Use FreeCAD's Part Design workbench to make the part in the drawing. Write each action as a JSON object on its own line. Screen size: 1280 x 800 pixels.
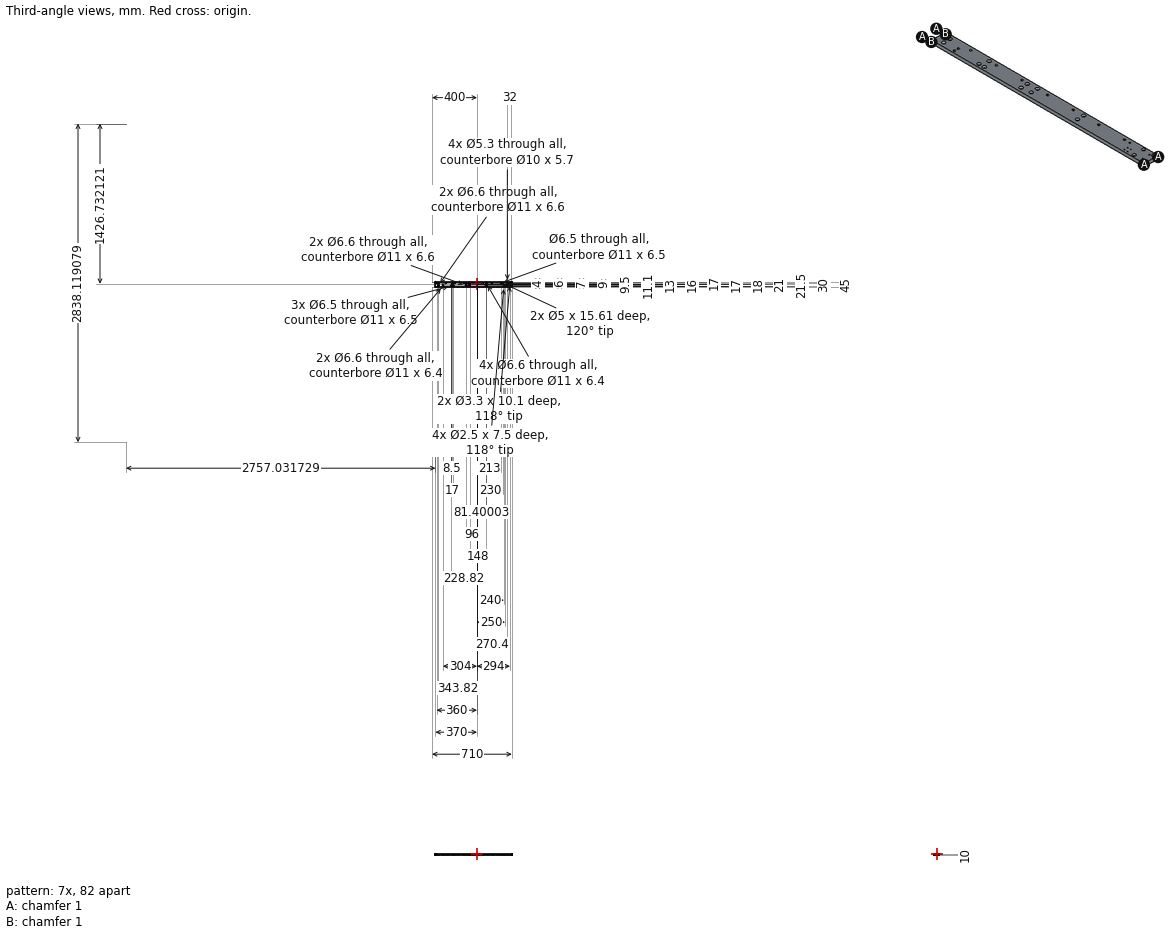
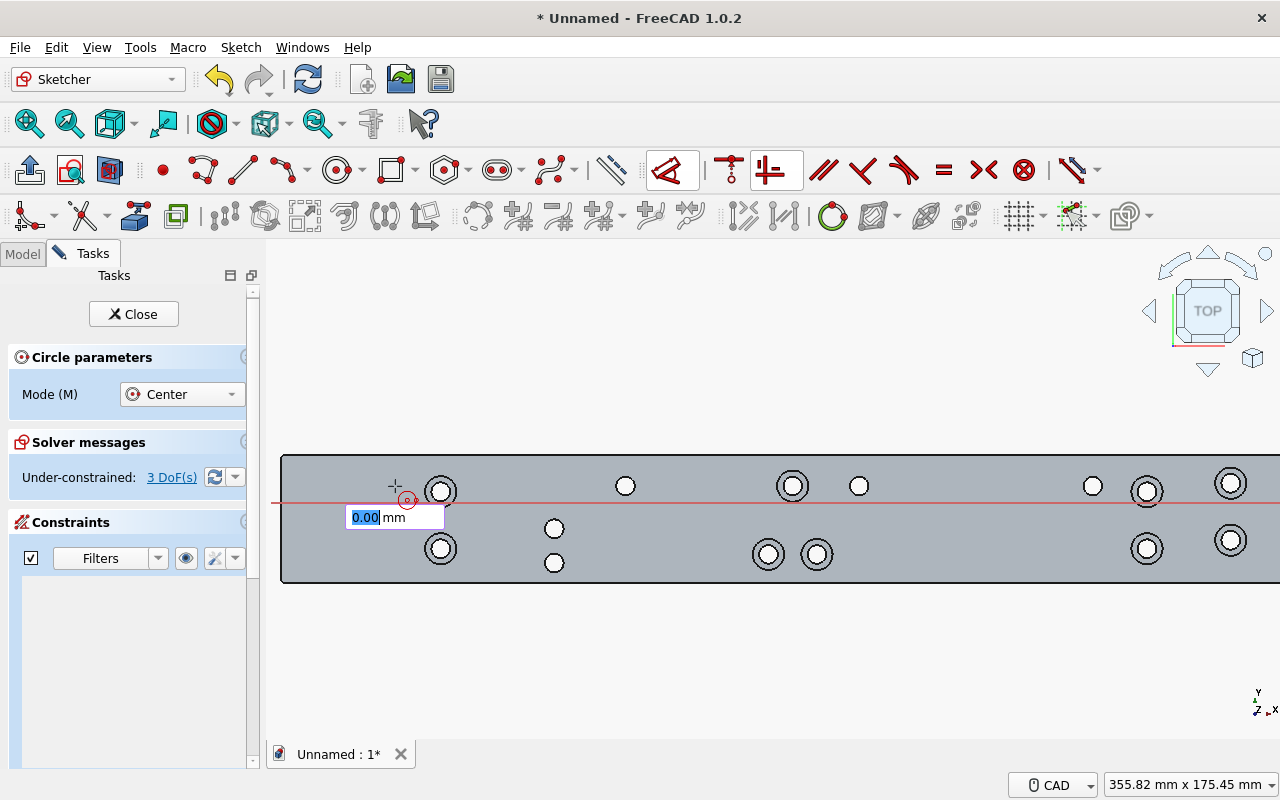
{"action": "scroll", "coordinate": [400, 481], "scroll_direction": "up", "scroll_amount": 5}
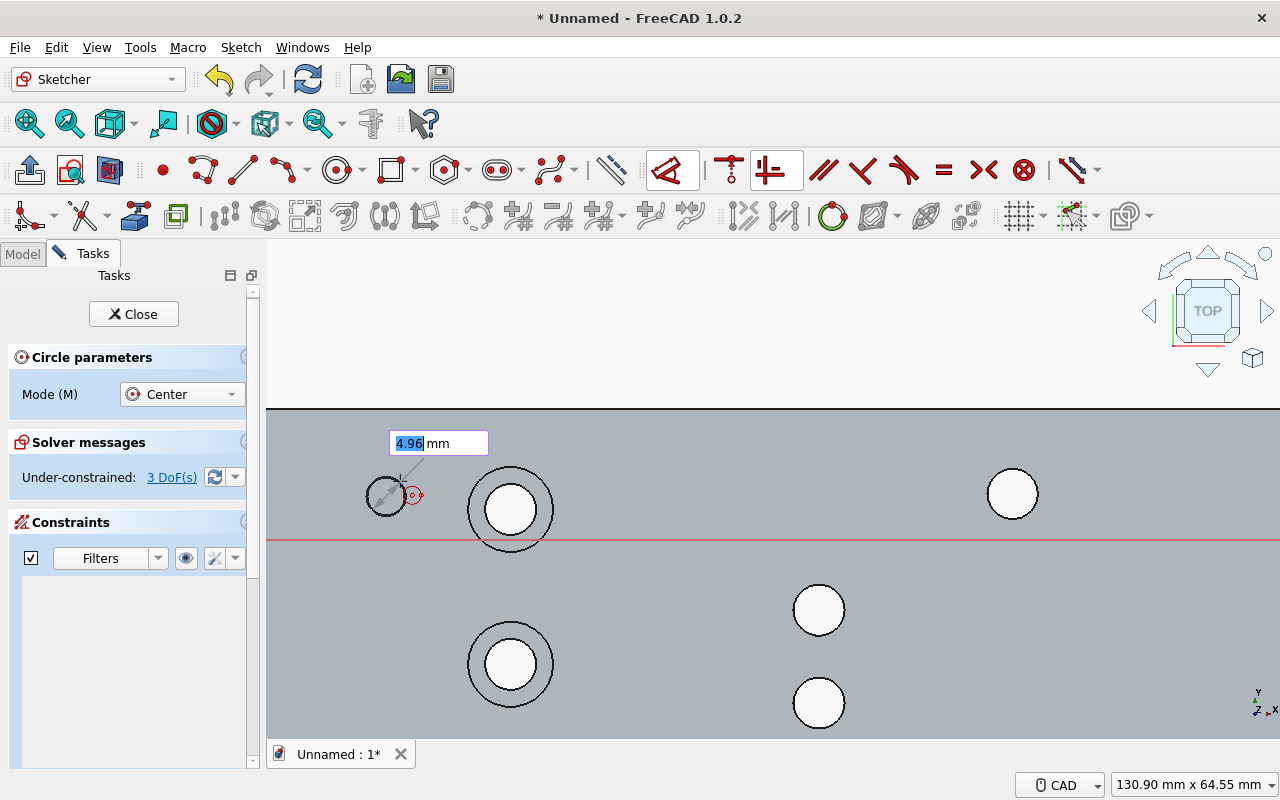
{"action": "left_click", "coordinate": [399, 480]}
{"action": "key", "text": "Escape"}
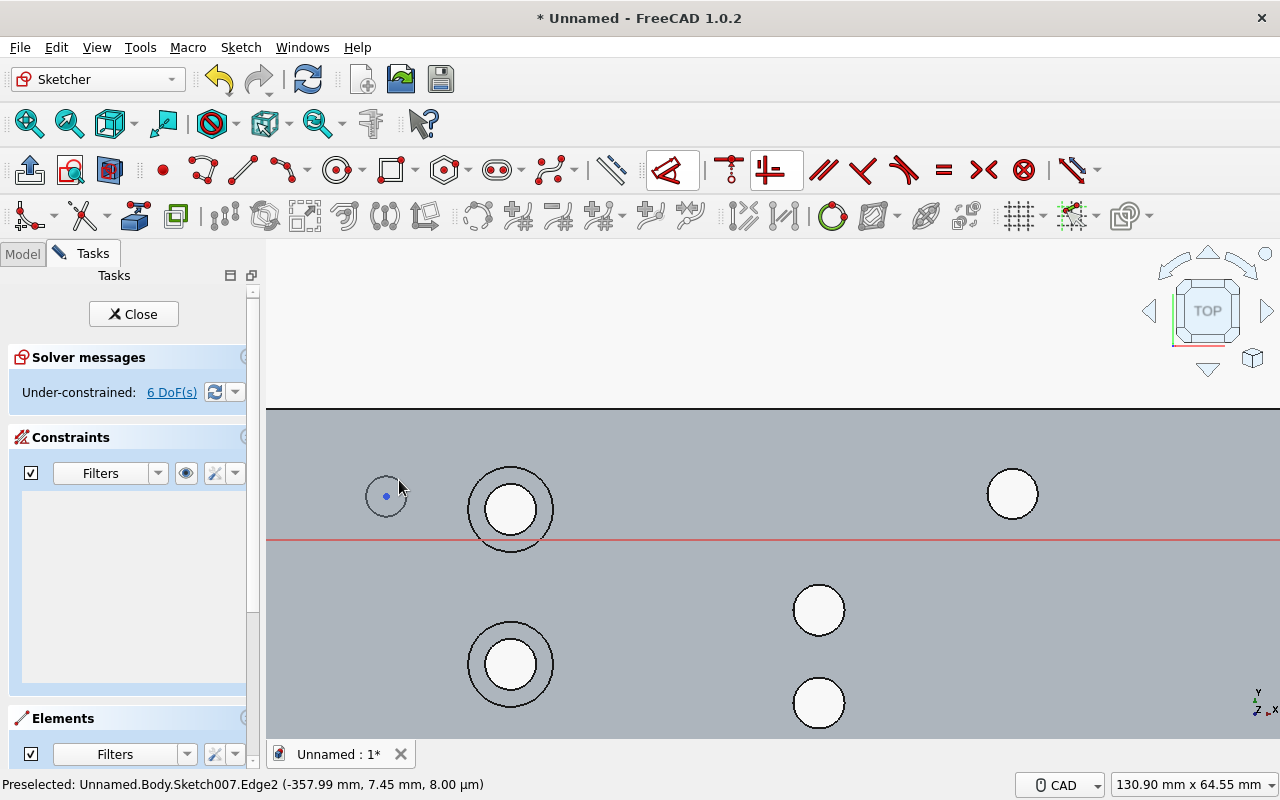
{"action": "scroll", "coordinate": [397, 486], "scroll_direction": "down", "scroll_amount": 10}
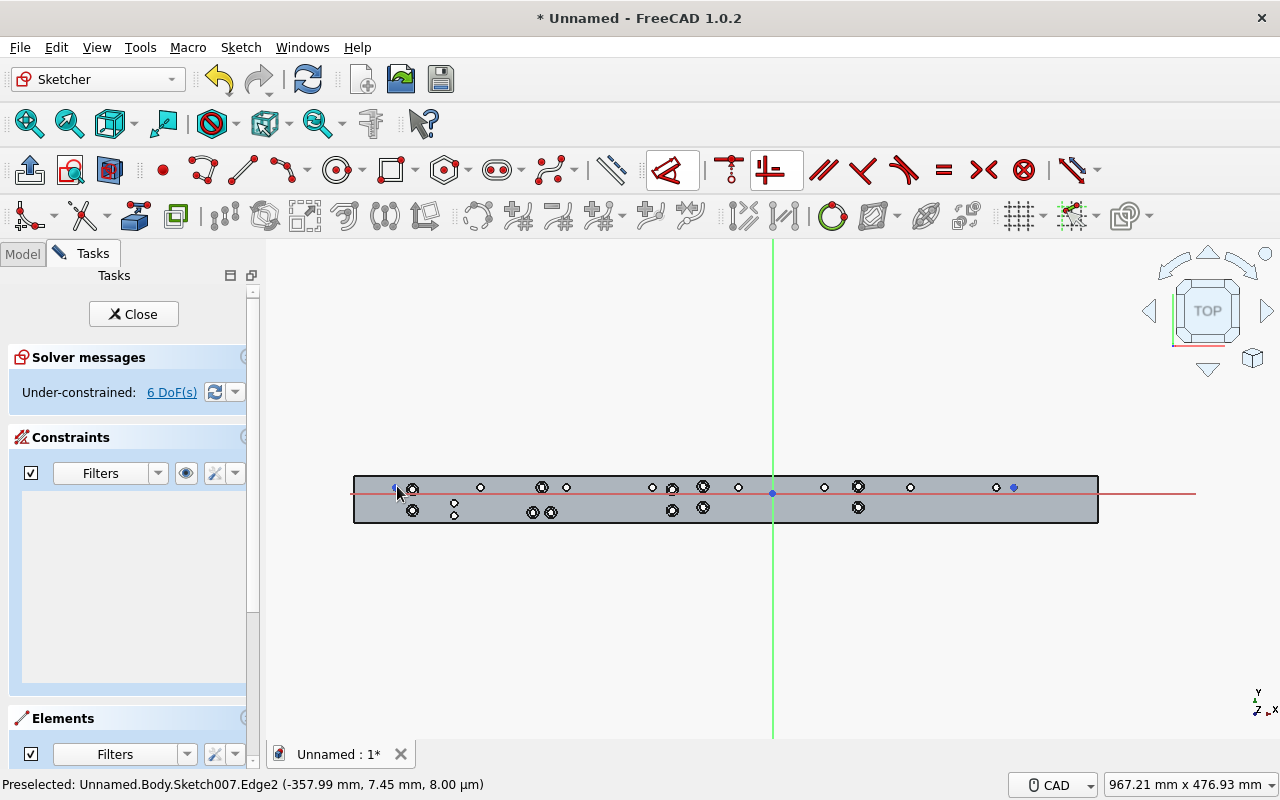
{"action": "scroll", "coordinate": [1016, 486], "scroll_direction": "up", "scroll_amount": 8}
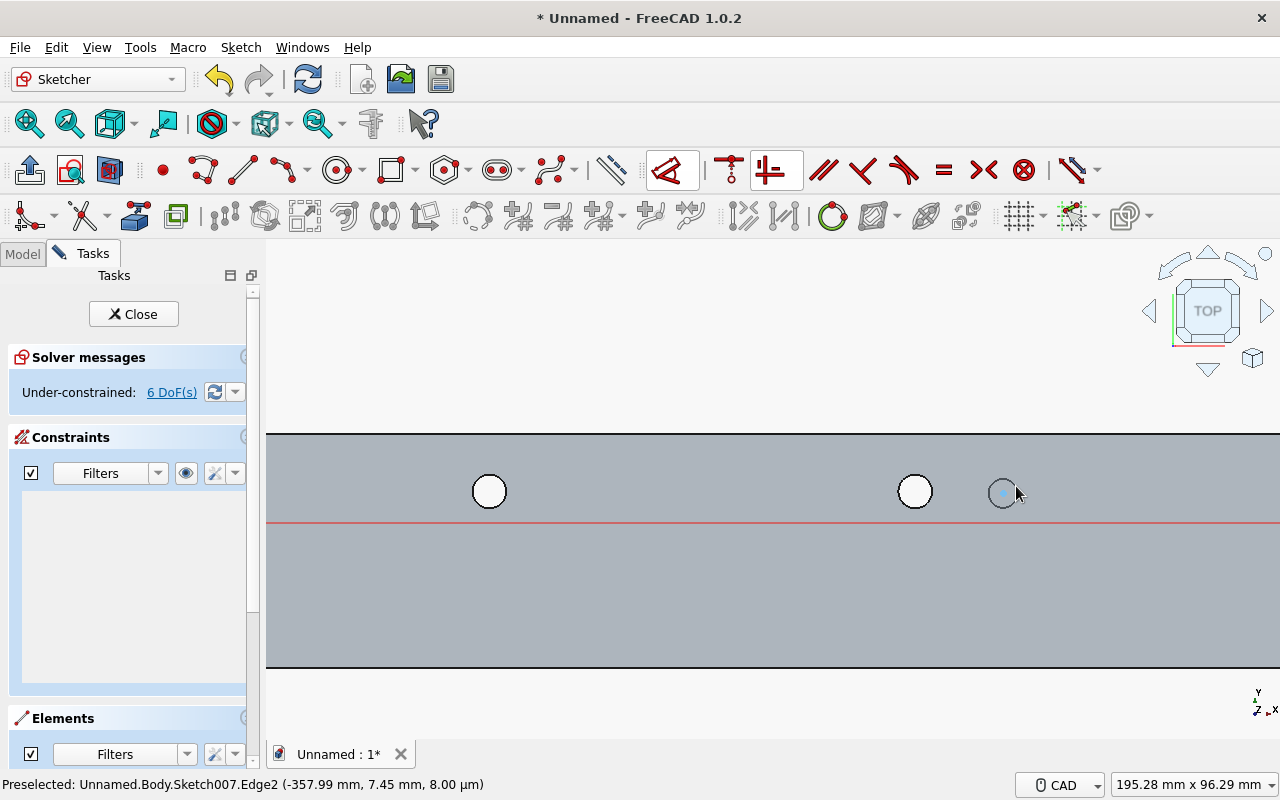
{"action": "left_click", "coordinate": [1013, 483]}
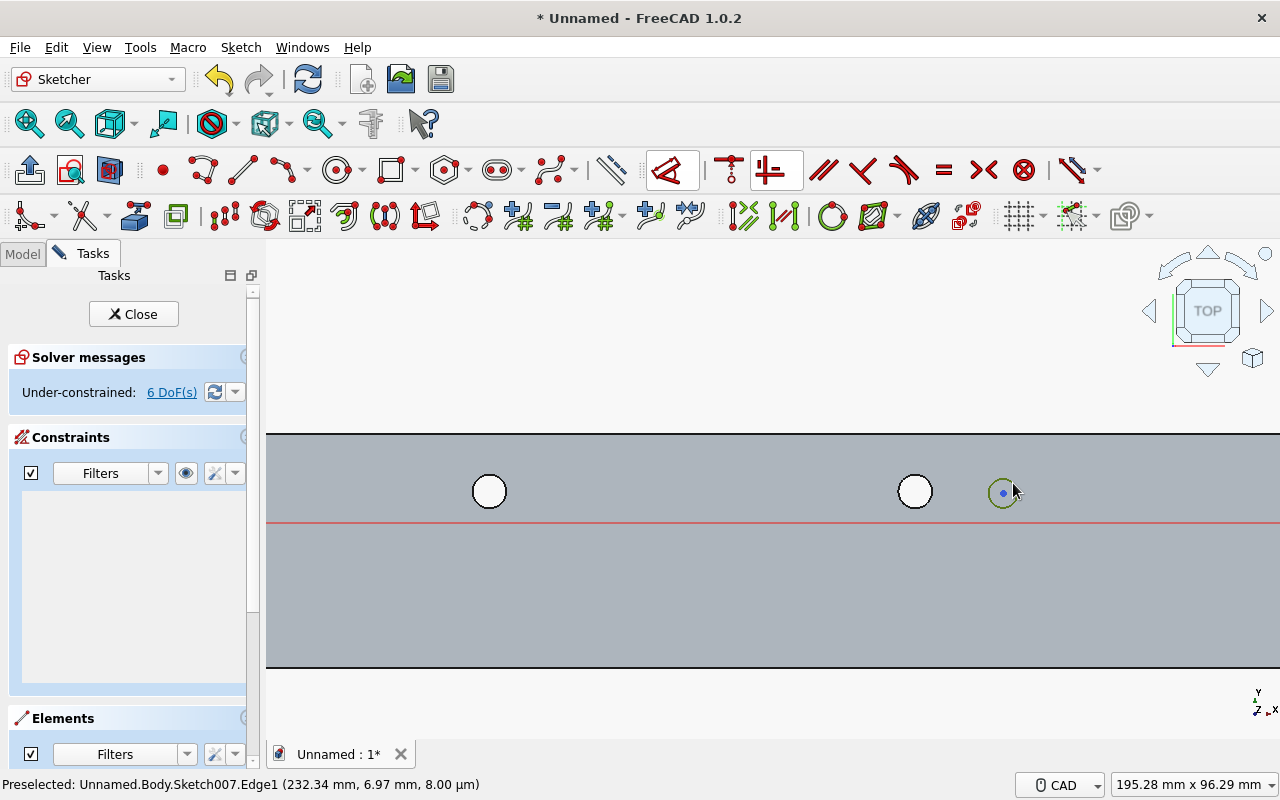
{"action": "scroll", "coordinate": [1016, 486], "scroll_direction": "down", "scroll_amount": 8}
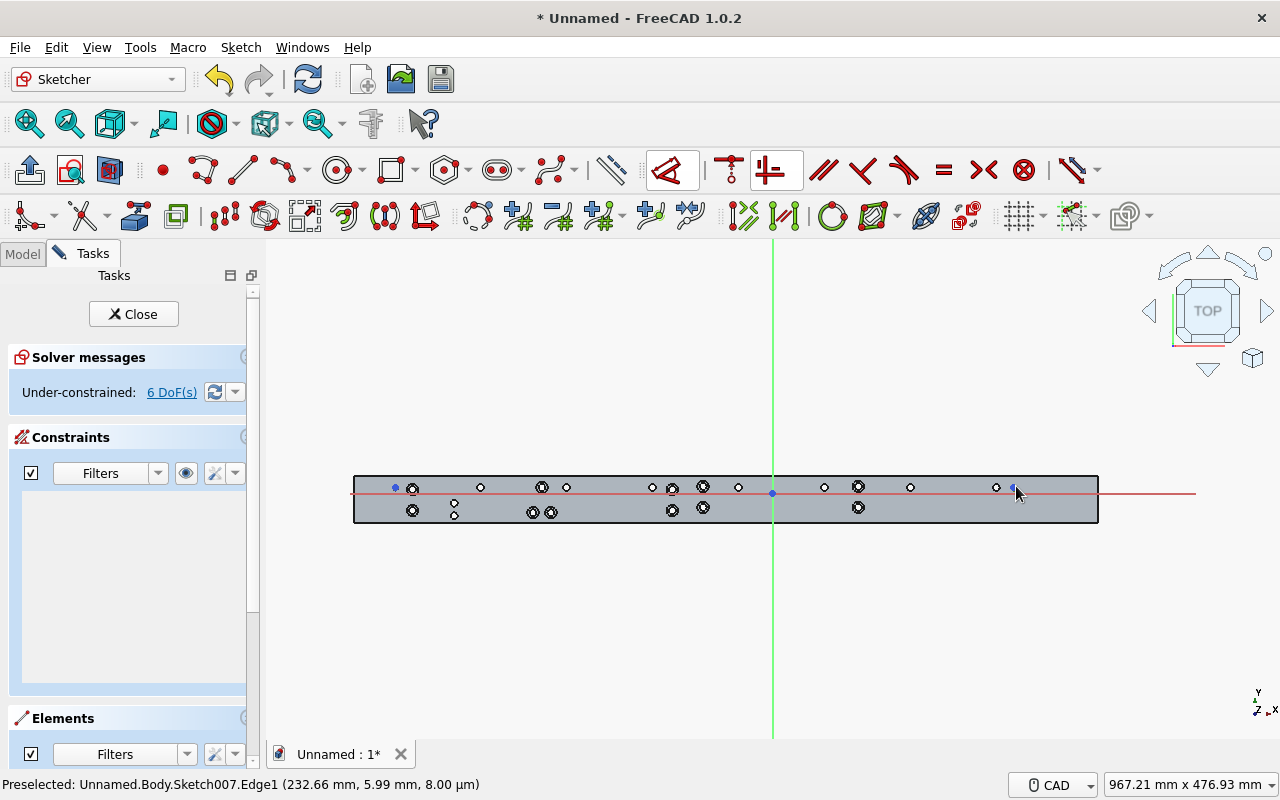
{"action": "scroll", "coordinate": [398, 486], "scroll_direction": "up", "scroll_amount": 9}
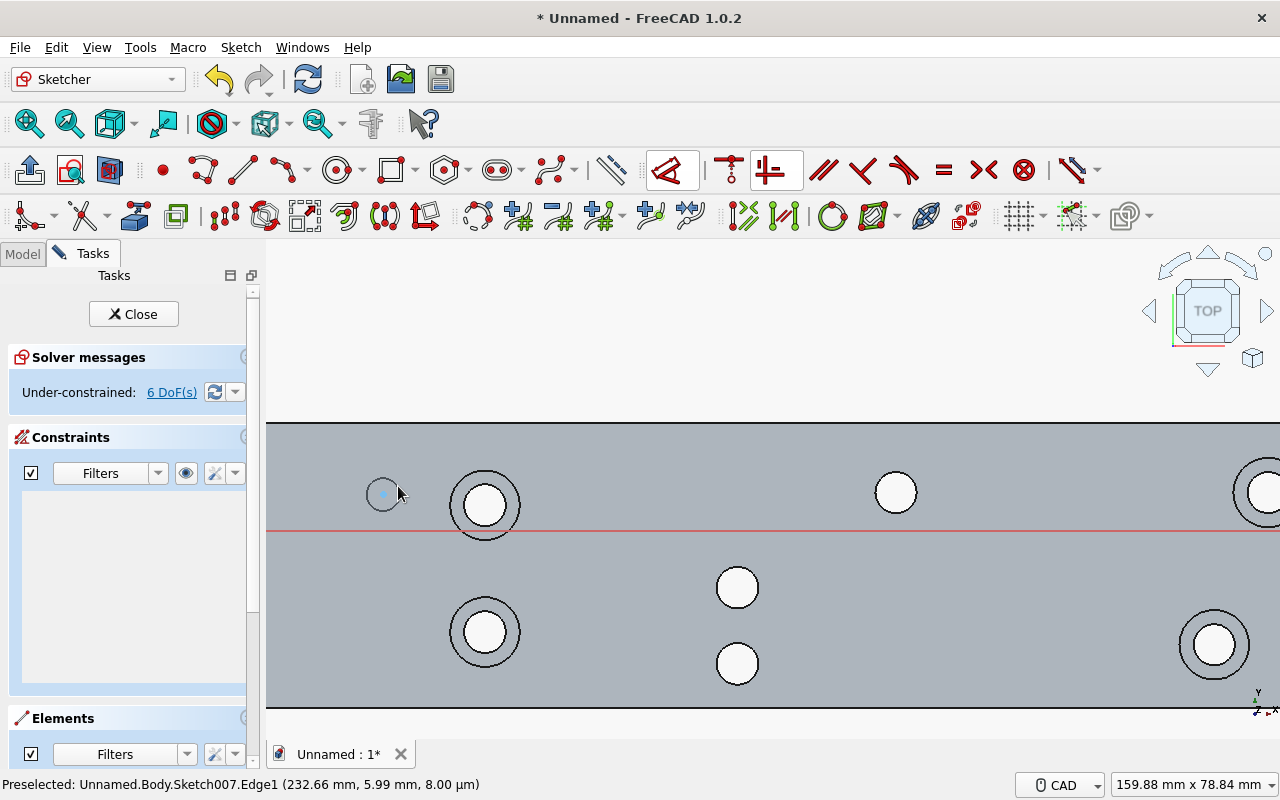
{"action": "left_click", "coordinate": [395, 483]}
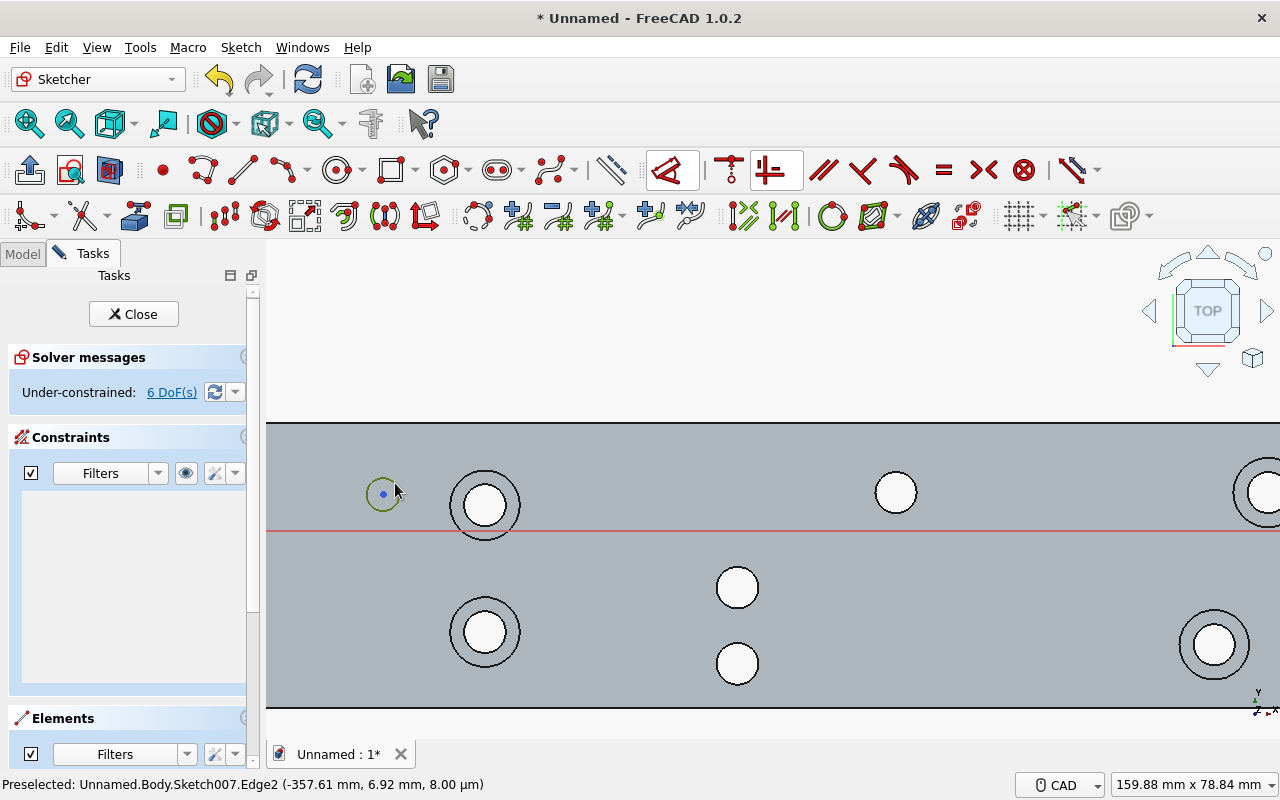
{"action": "left_click", "coordinate": [944, 170]}